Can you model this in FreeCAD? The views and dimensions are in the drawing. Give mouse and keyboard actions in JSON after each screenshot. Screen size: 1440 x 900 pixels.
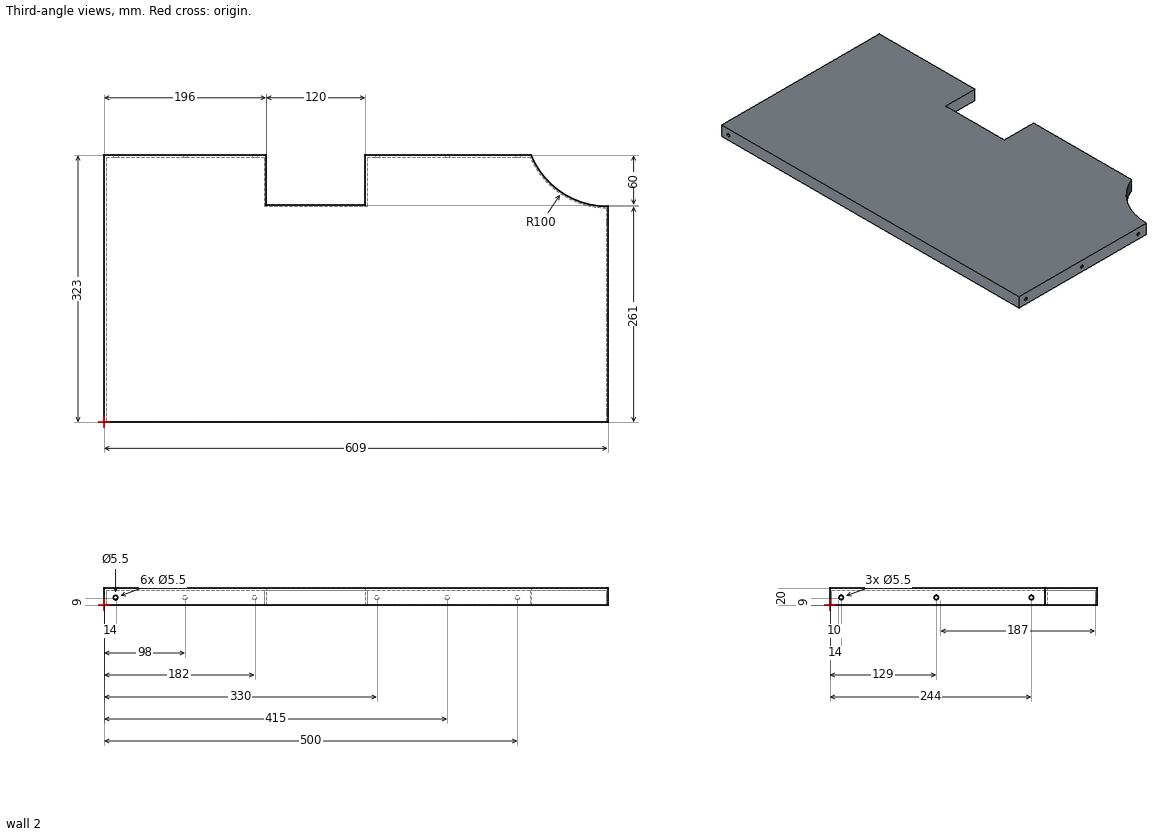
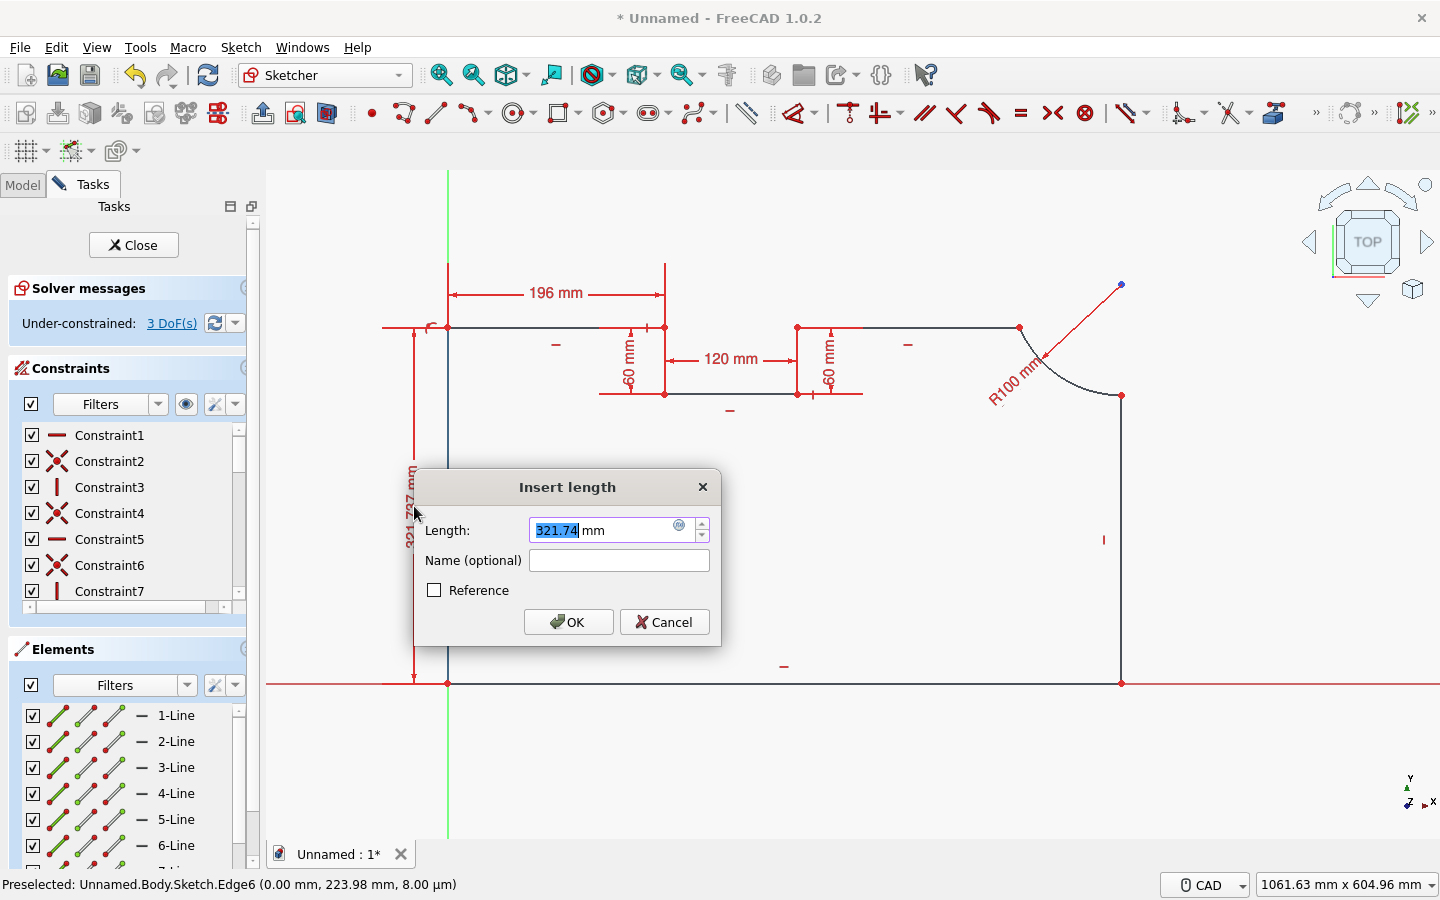
{"action": "type", "text": "323"}
{"action": "key", "text": "Return"}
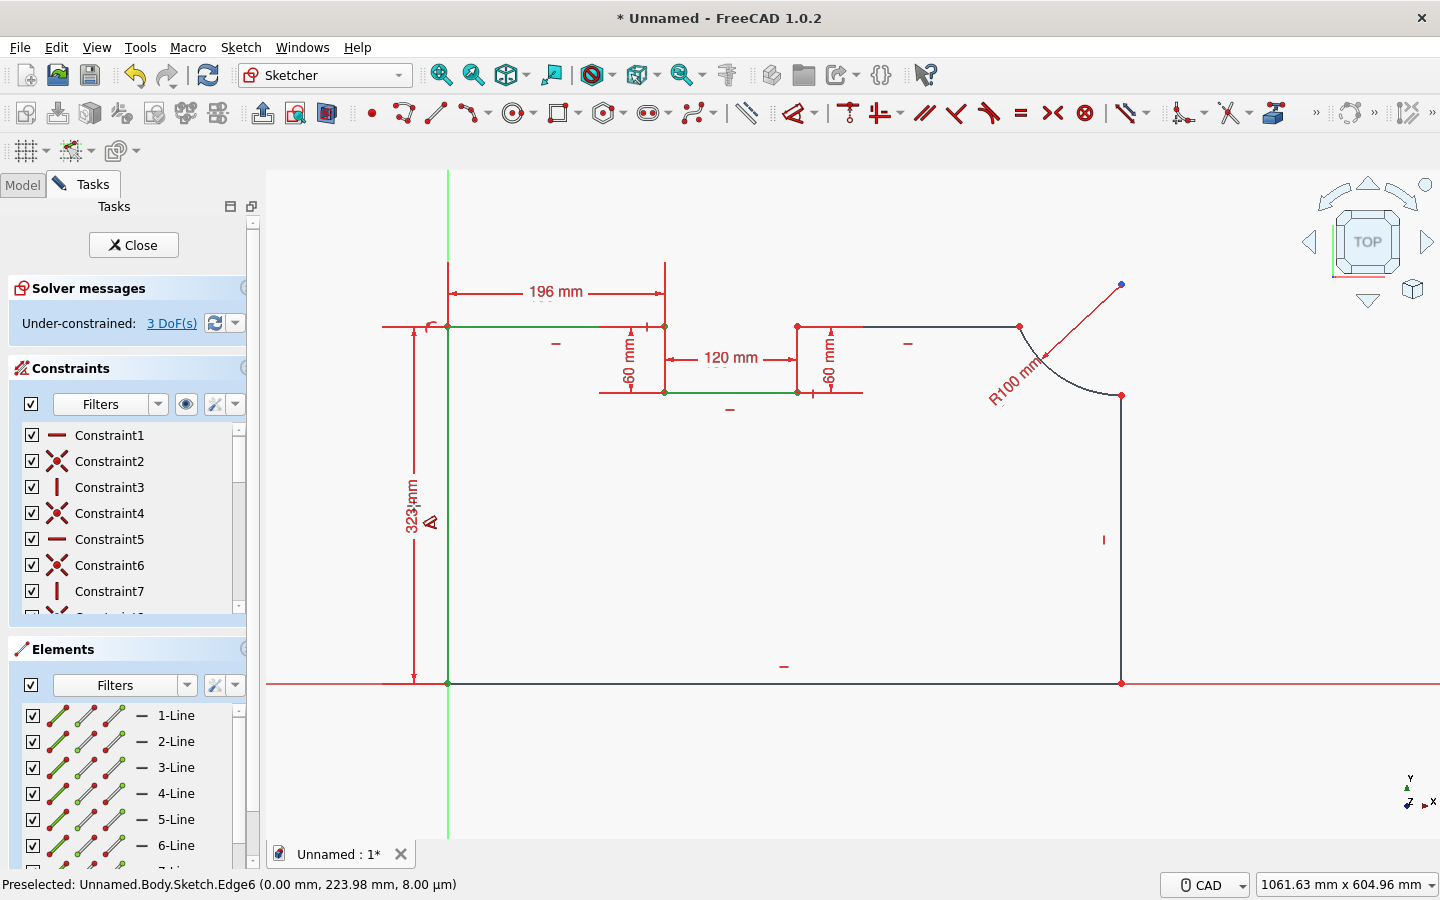
{"action": "left_click", "coordinate": [650, 684]}
{"action": "left_click", "coordinate": [784, 718]}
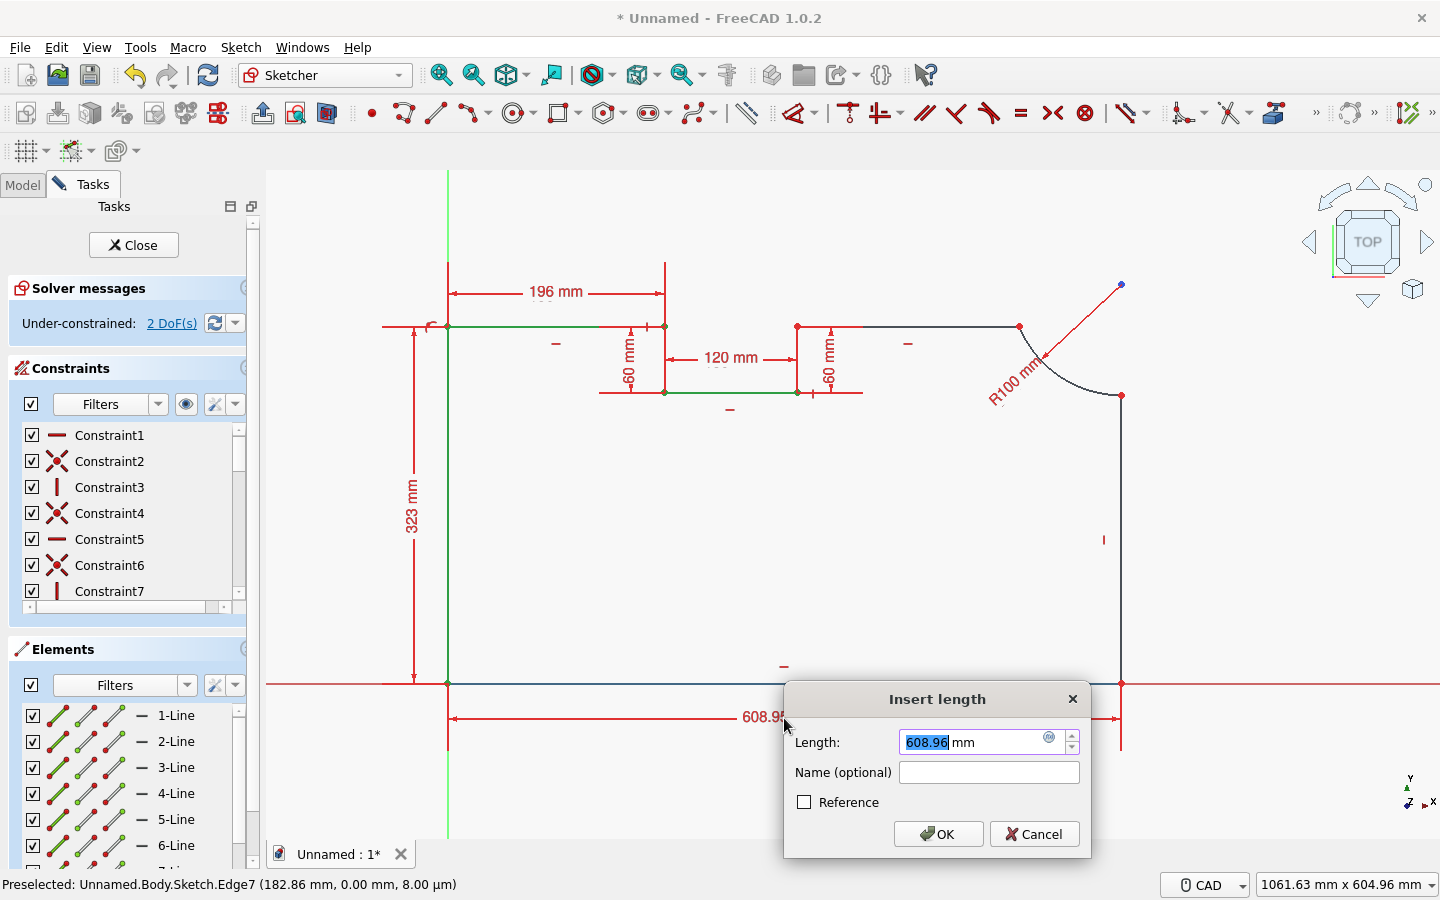
{"action": "type", "text": "609"}
{"action": "key", "text": "Return"}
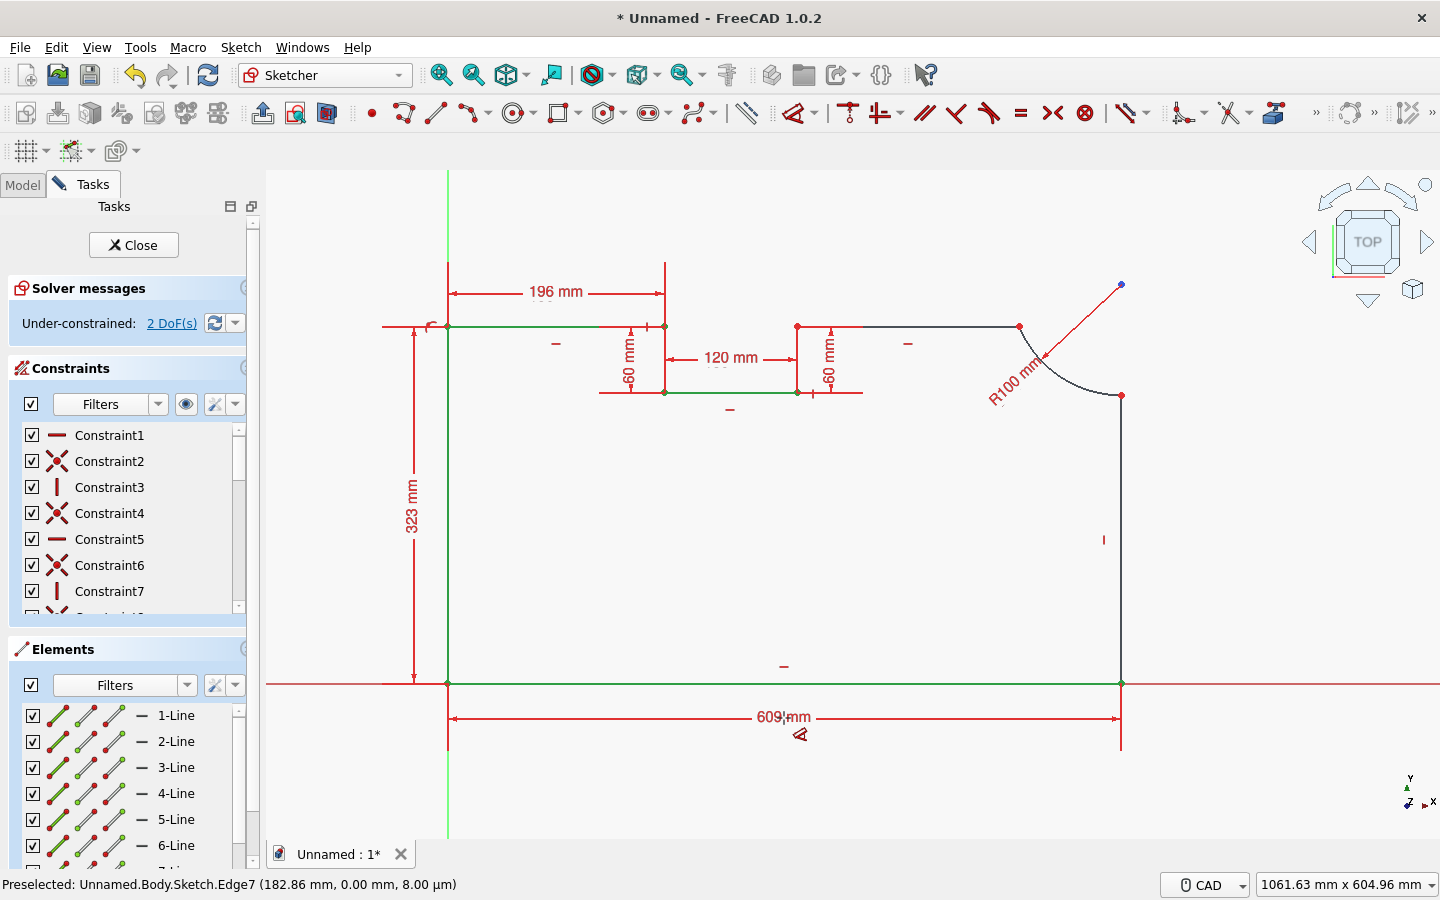
{"action": "left_click", "coordinate": [1121, 597]}
{"action": "left_click", "coordinate": [1155, 540]}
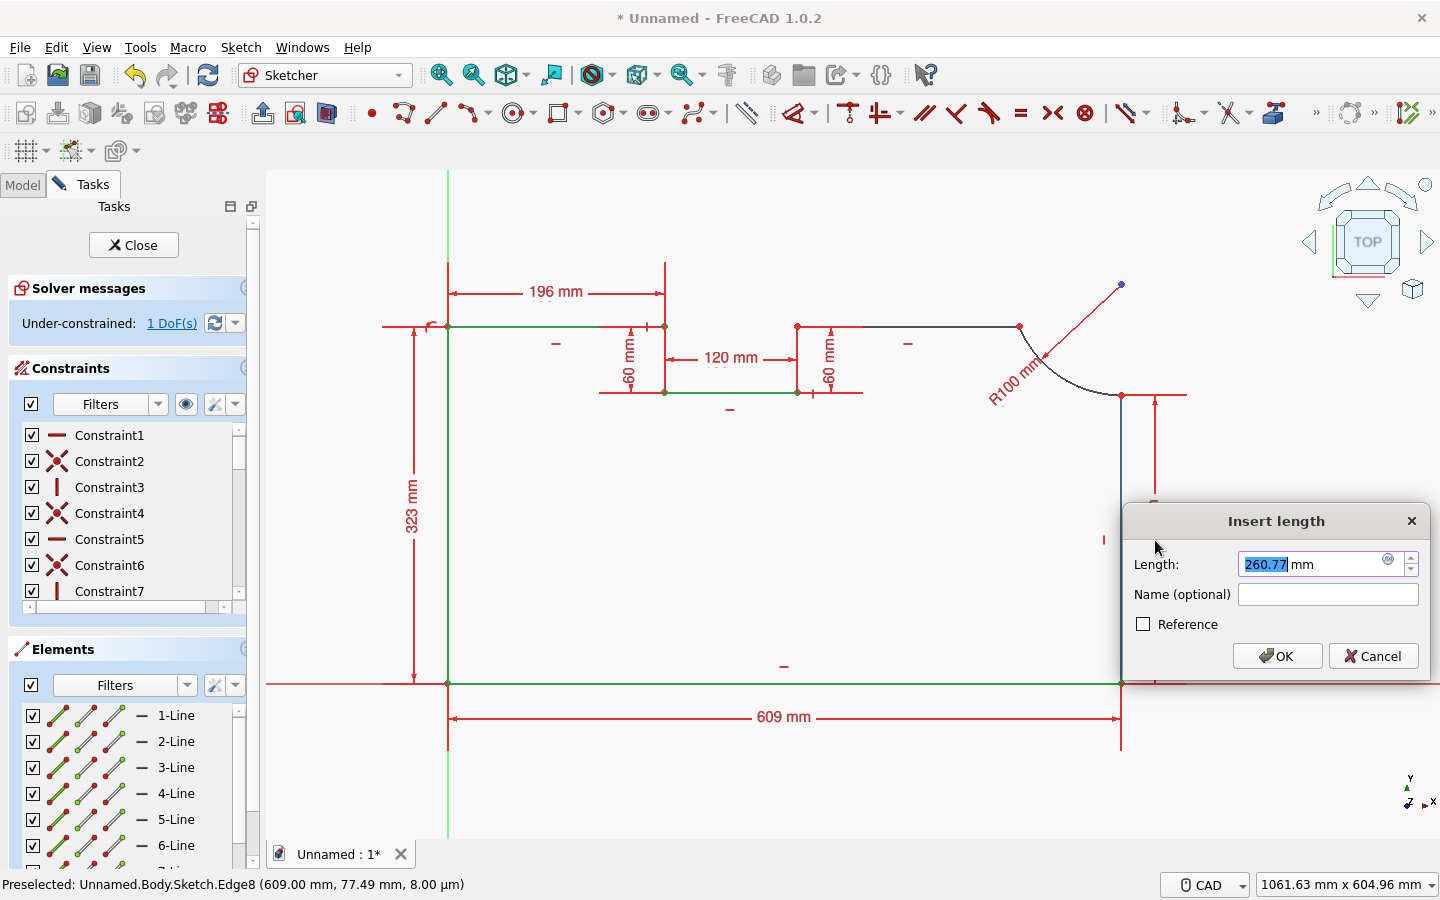
{"action": "type", "text": "261"}
{"action": "key", "text": "Return"}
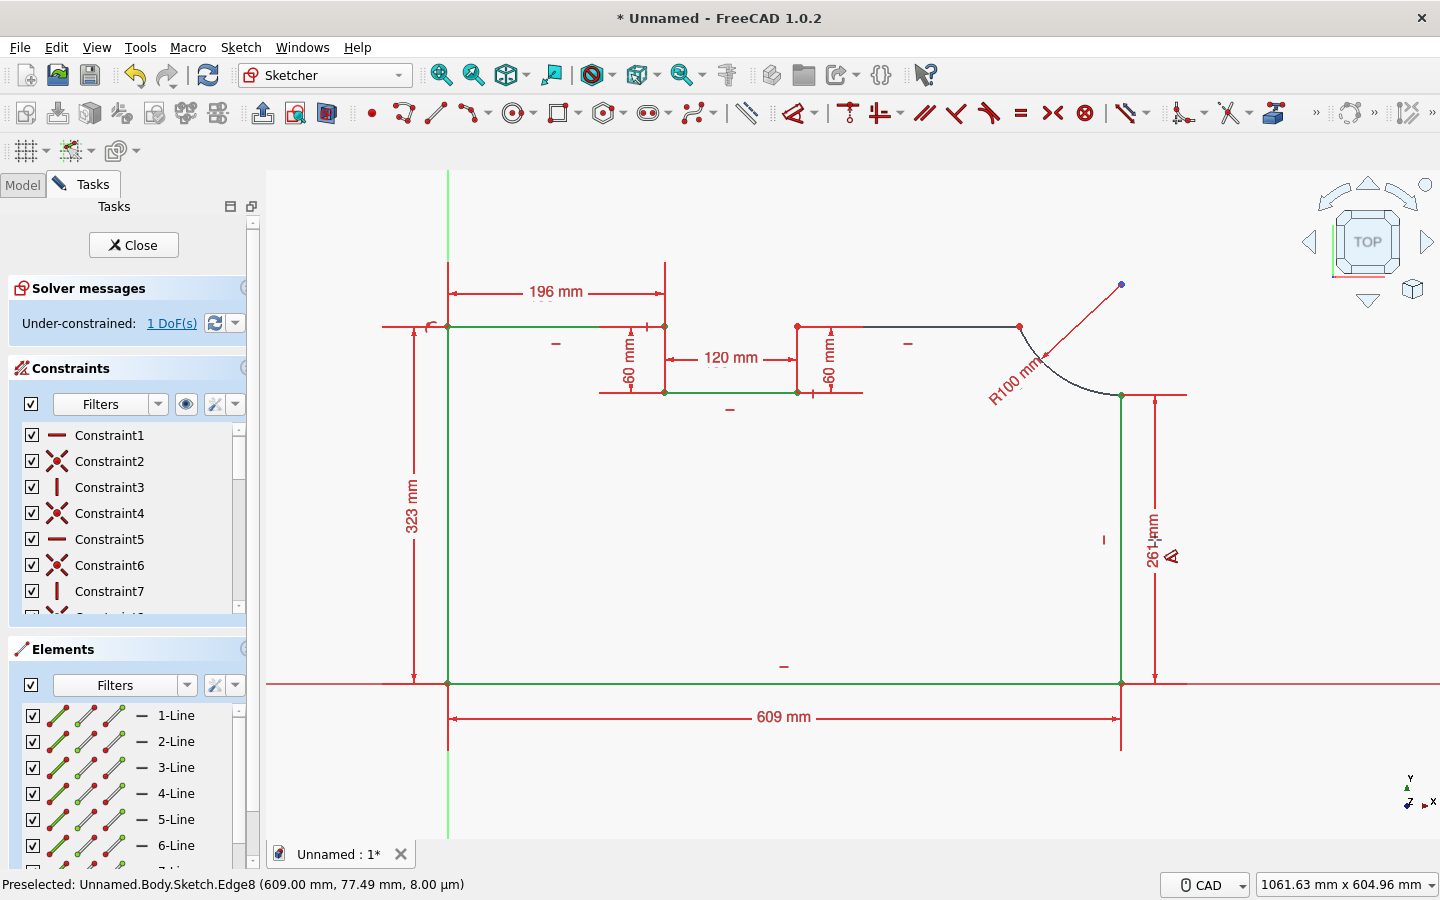
{"action": "left_click", "coordinate": [1122, 284]}
{"action": "left_click", "coordinate": [785, 250]}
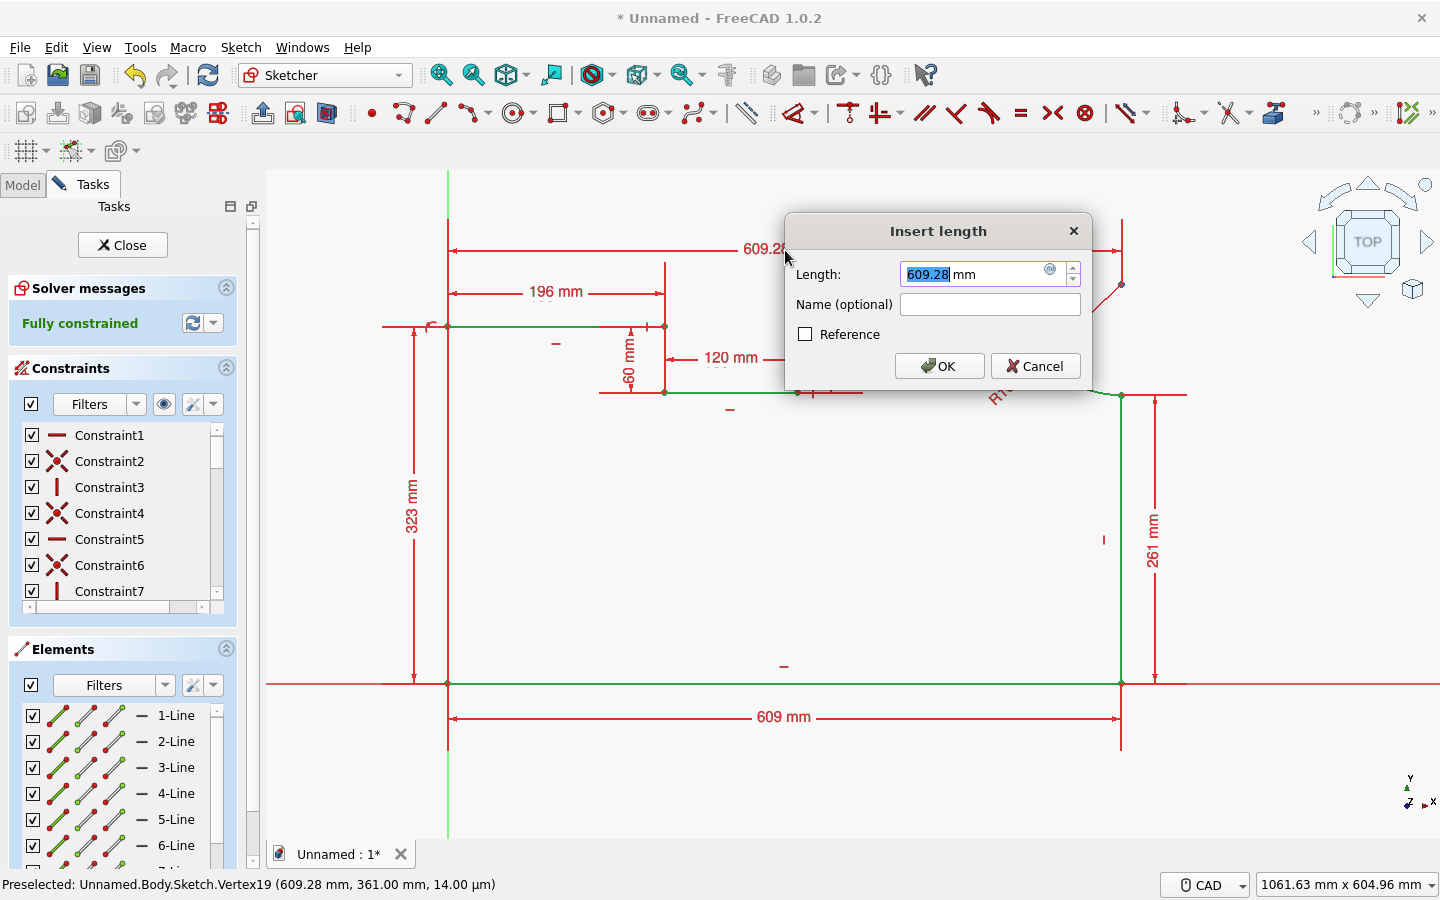
{"action": "type", "text": "609"}
{"action": "key", "text": "Return"}
{"action": "key", "text": "Escape"}